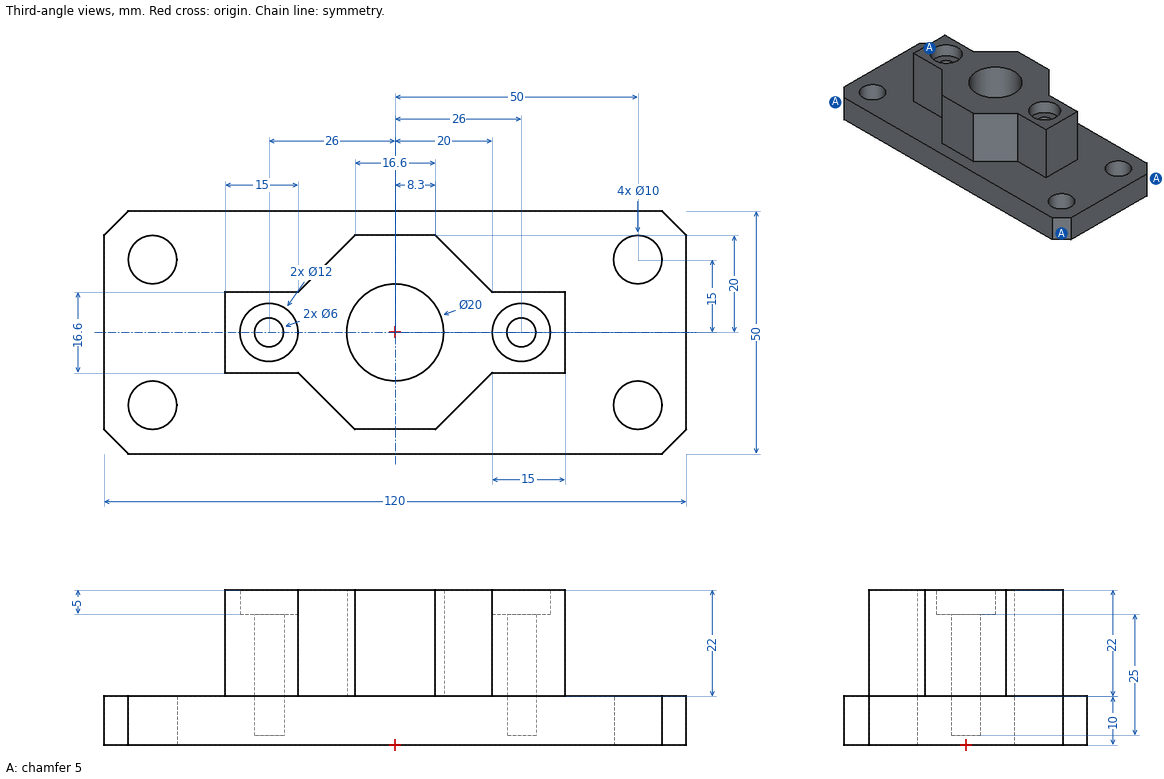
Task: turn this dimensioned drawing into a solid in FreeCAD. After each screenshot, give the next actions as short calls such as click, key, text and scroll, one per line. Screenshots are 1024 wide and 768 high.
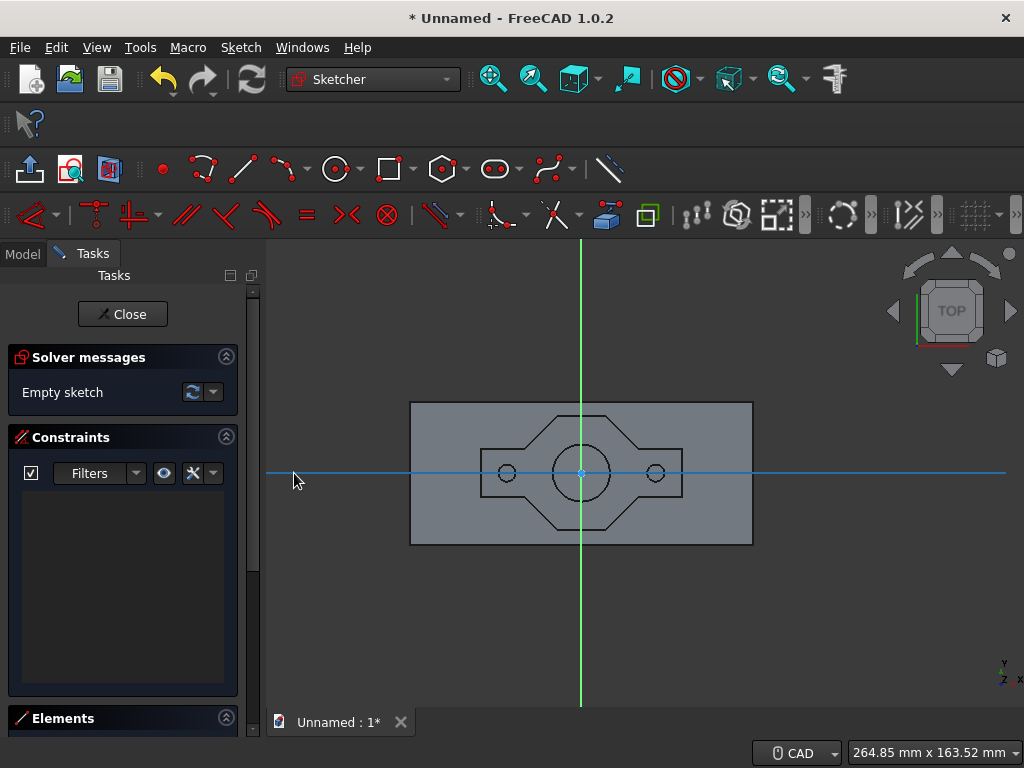
click(336, 170)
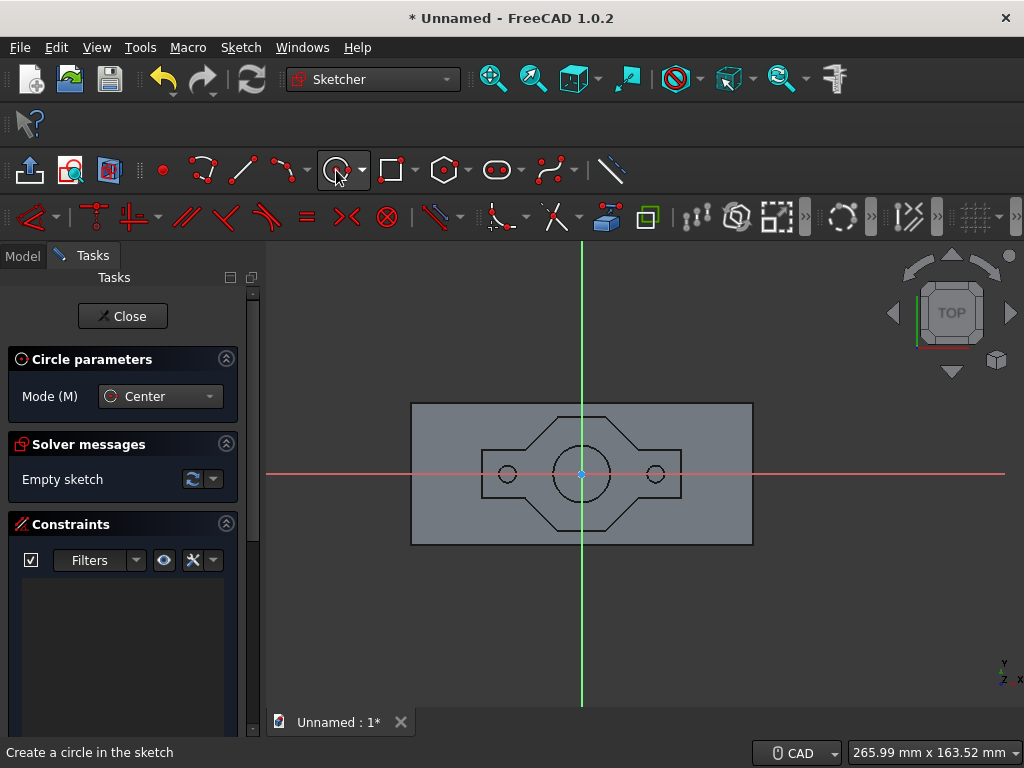
scroll(724, 431, up, 3)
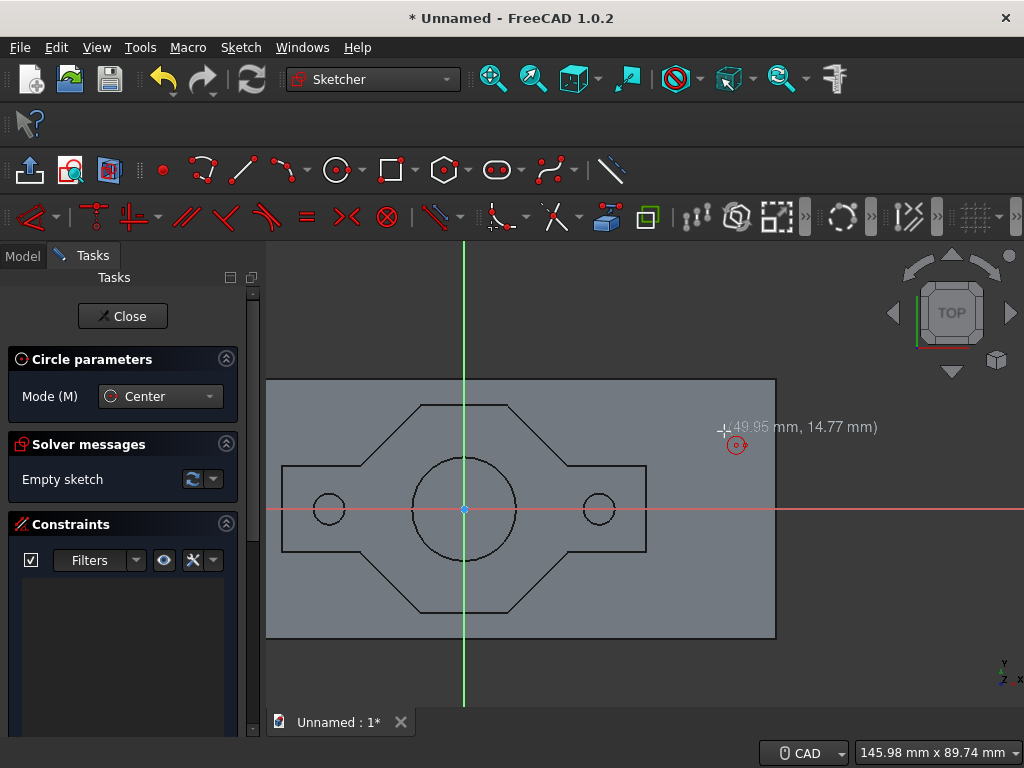
click(724, 431)
click(742, 413)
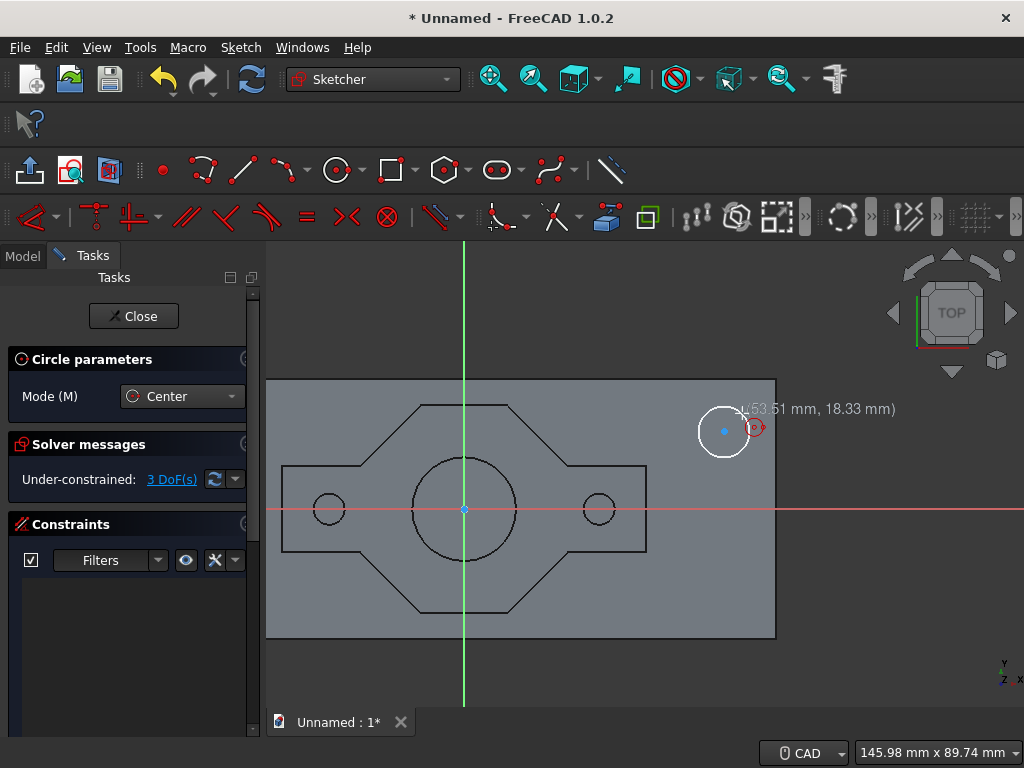
click(724, 587)
click(742, 569)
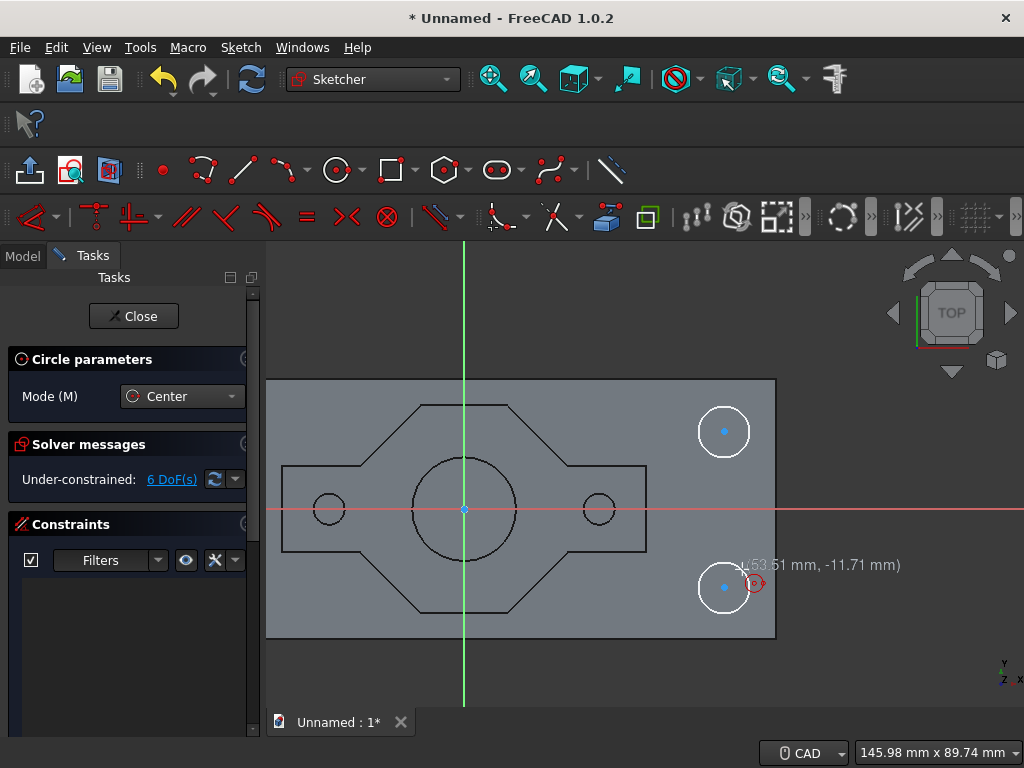
scroll(805, 402, down, 2)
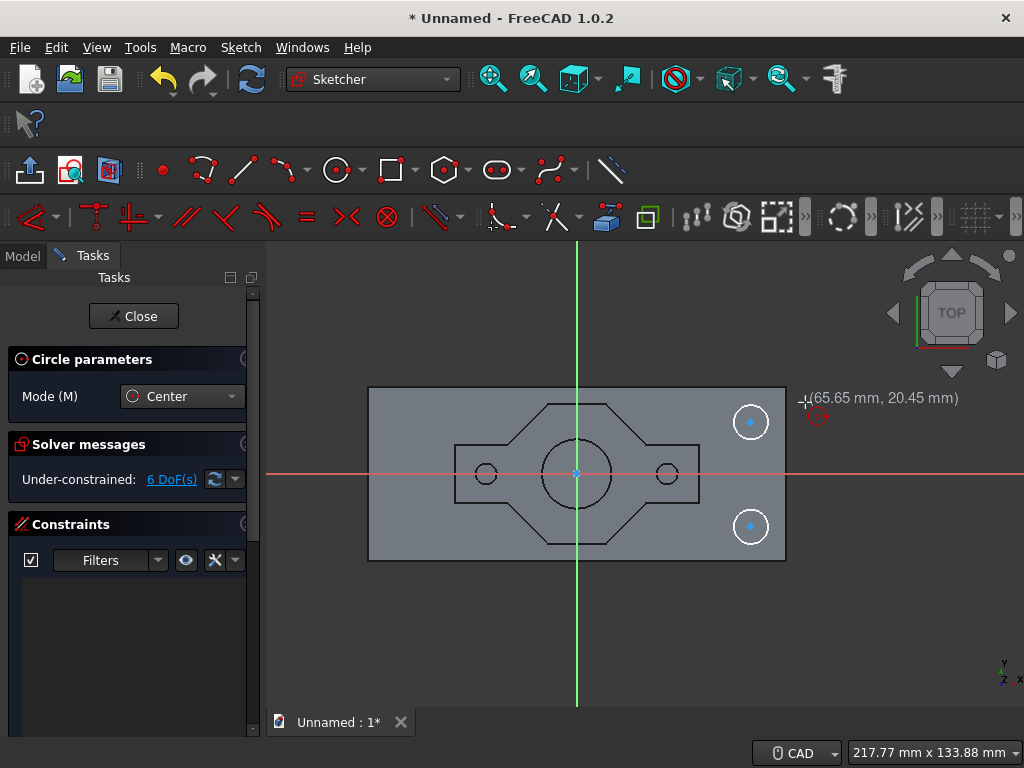
scroll(403, 422, up, 2)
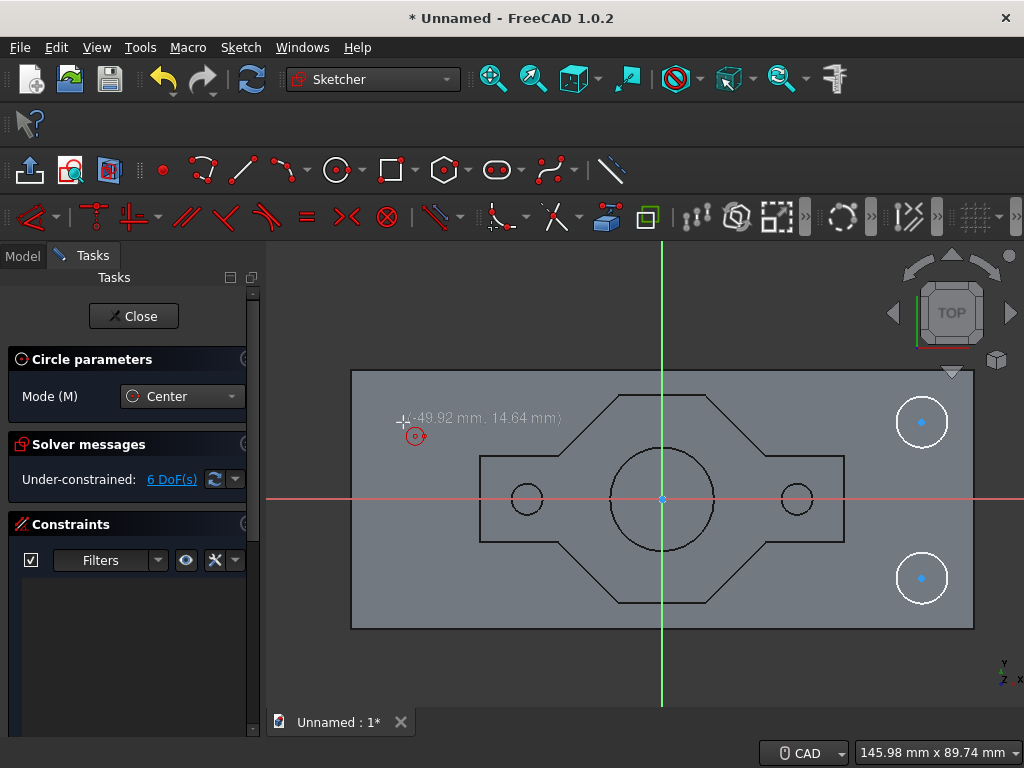
click(402, 421)
click(421, 403)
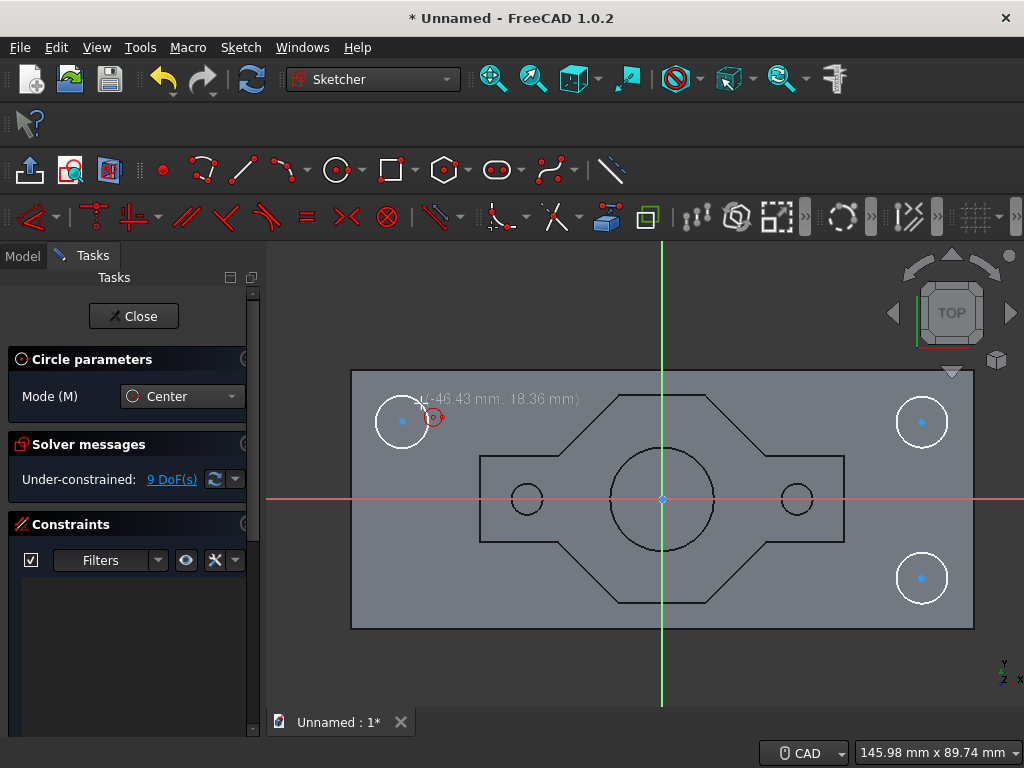
click(402, 577)
click(421, 559)
key(Escape)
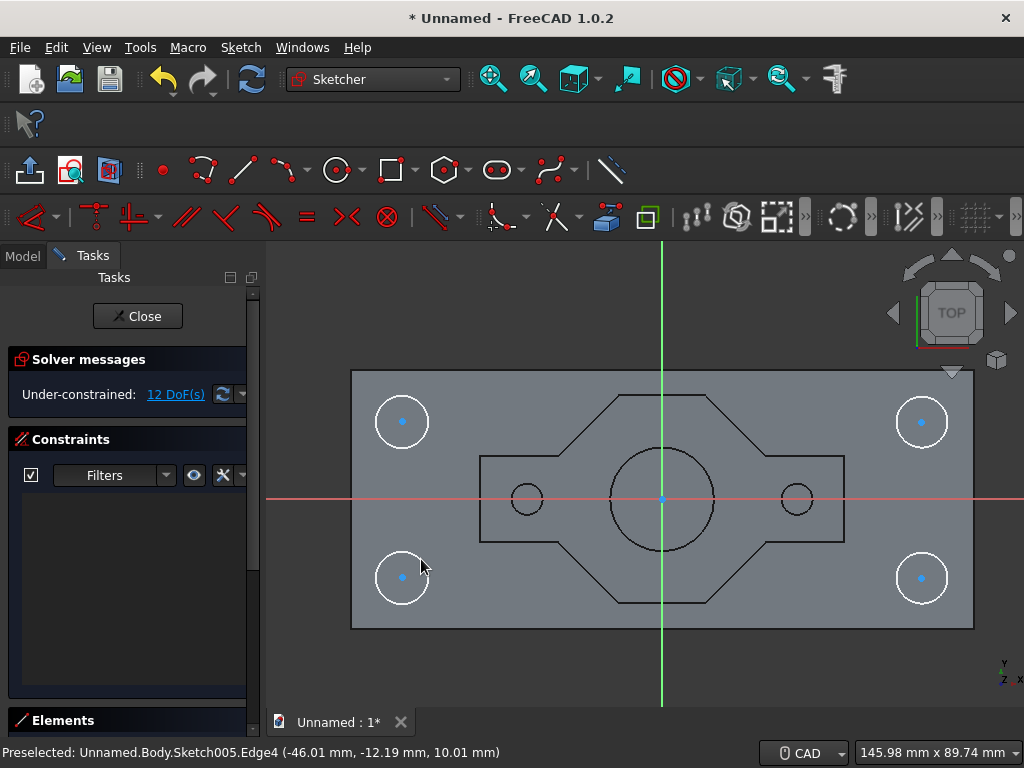
scroll(402, 423, down, 2)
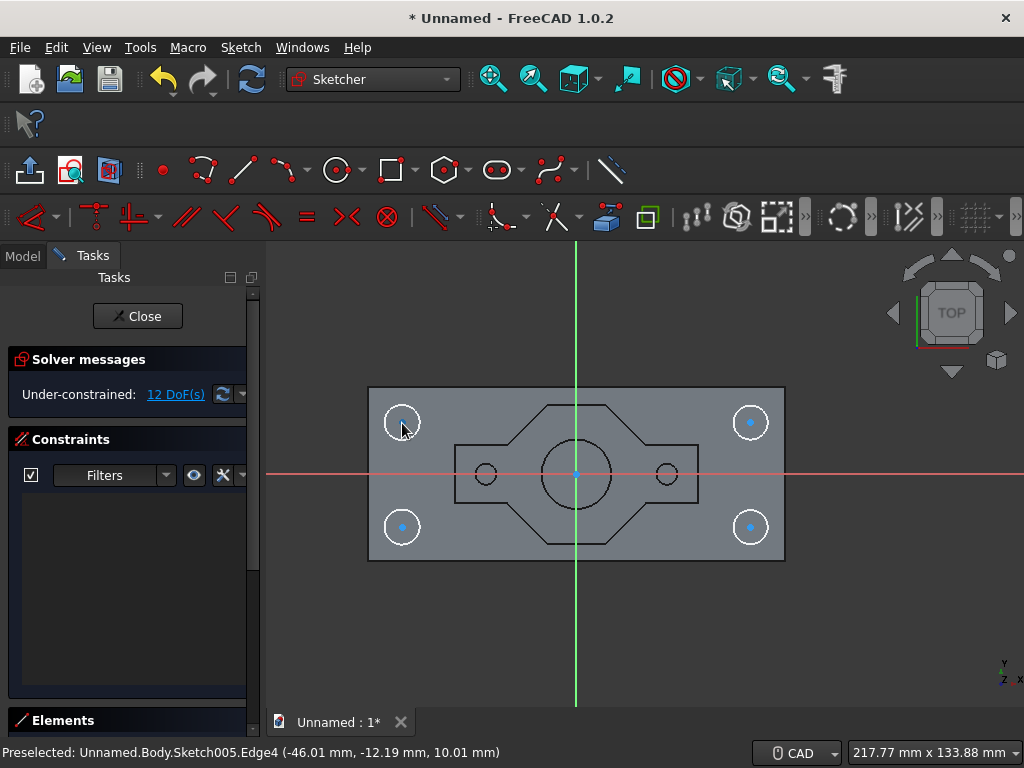
click(763, 410)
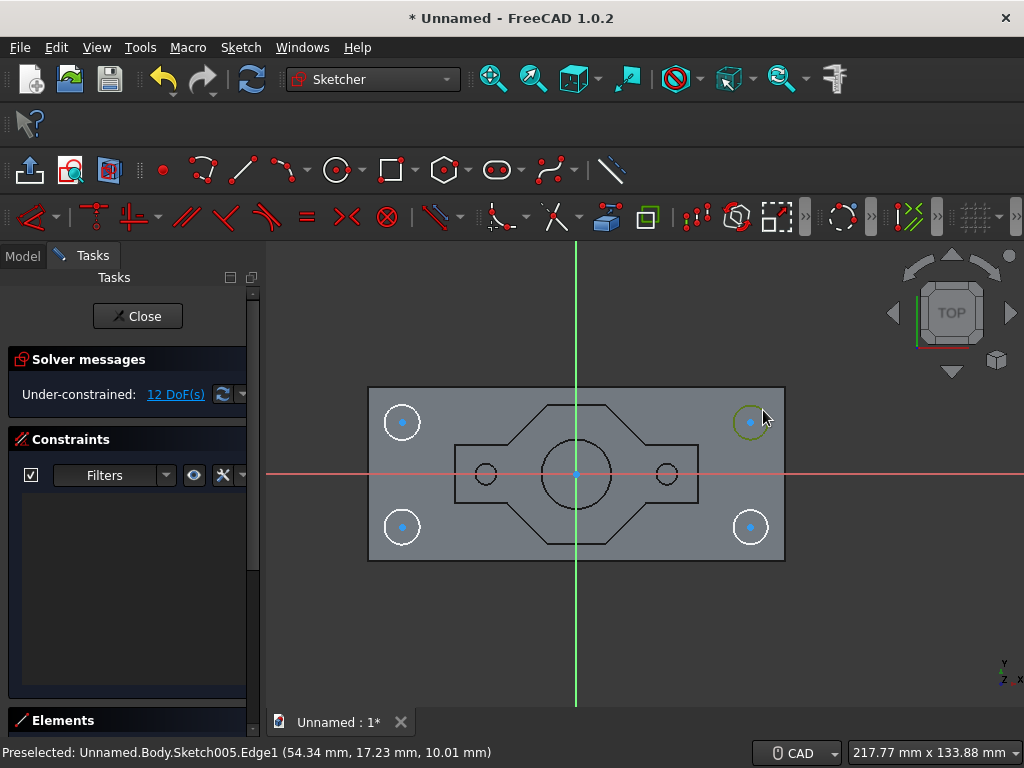
click(763, 515)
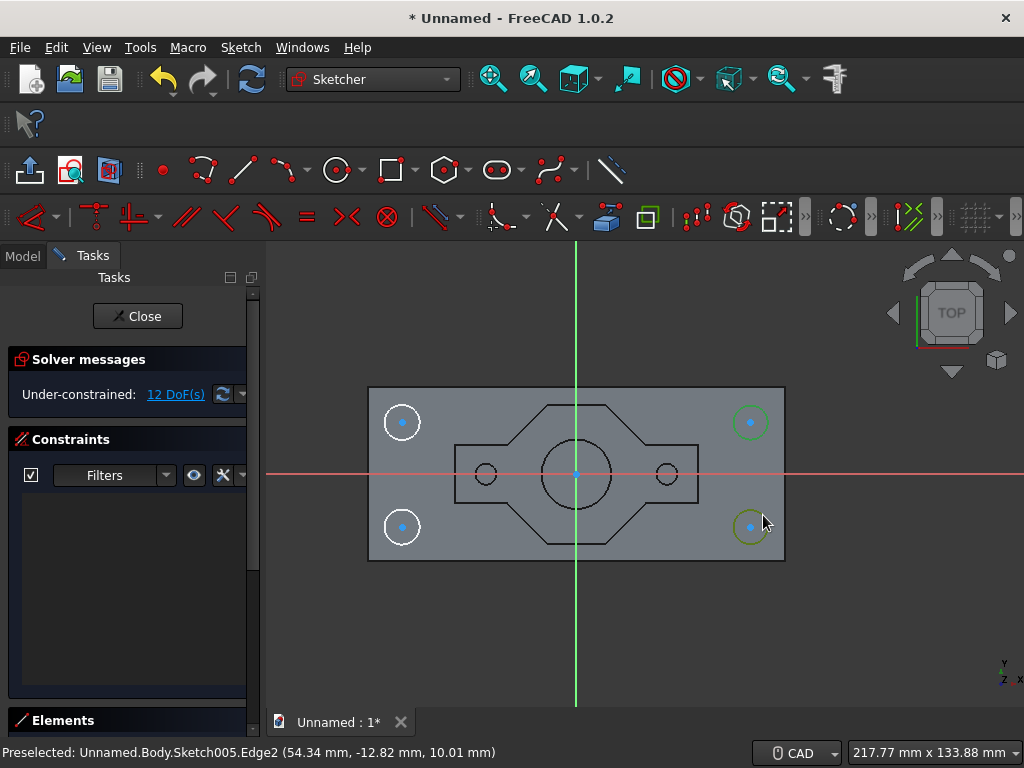
click(414, 410)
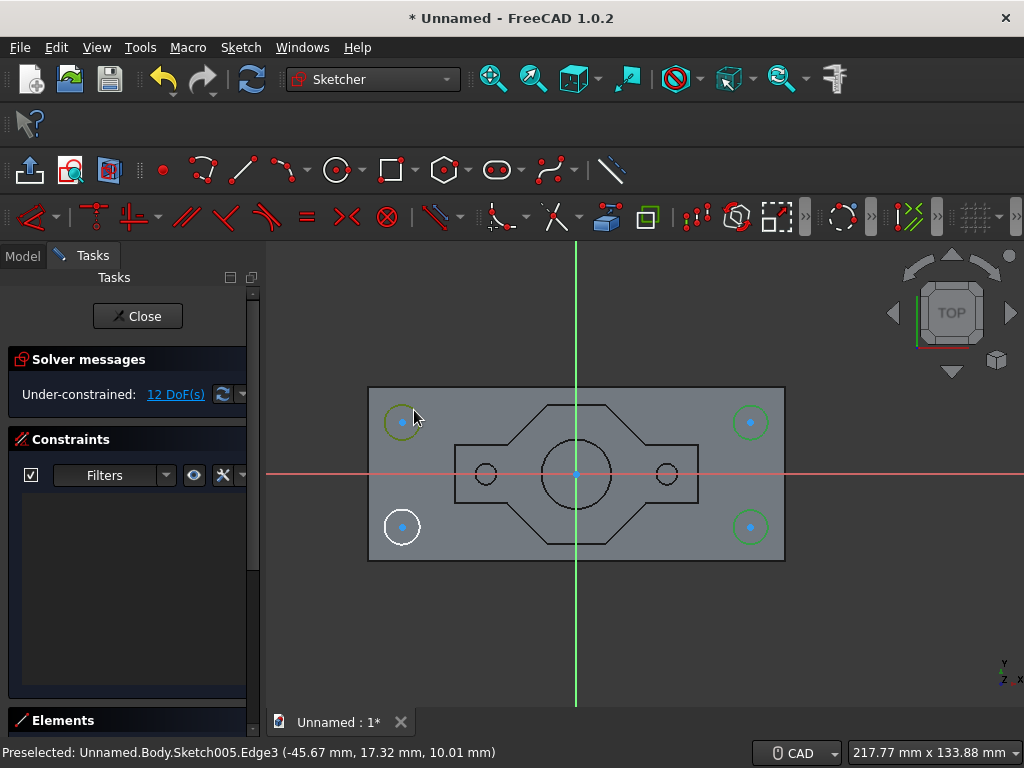
click(414, 515)